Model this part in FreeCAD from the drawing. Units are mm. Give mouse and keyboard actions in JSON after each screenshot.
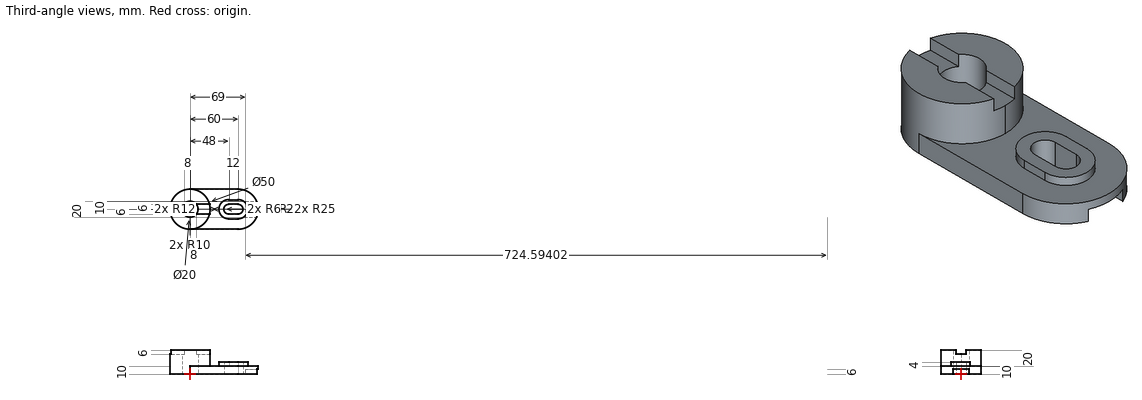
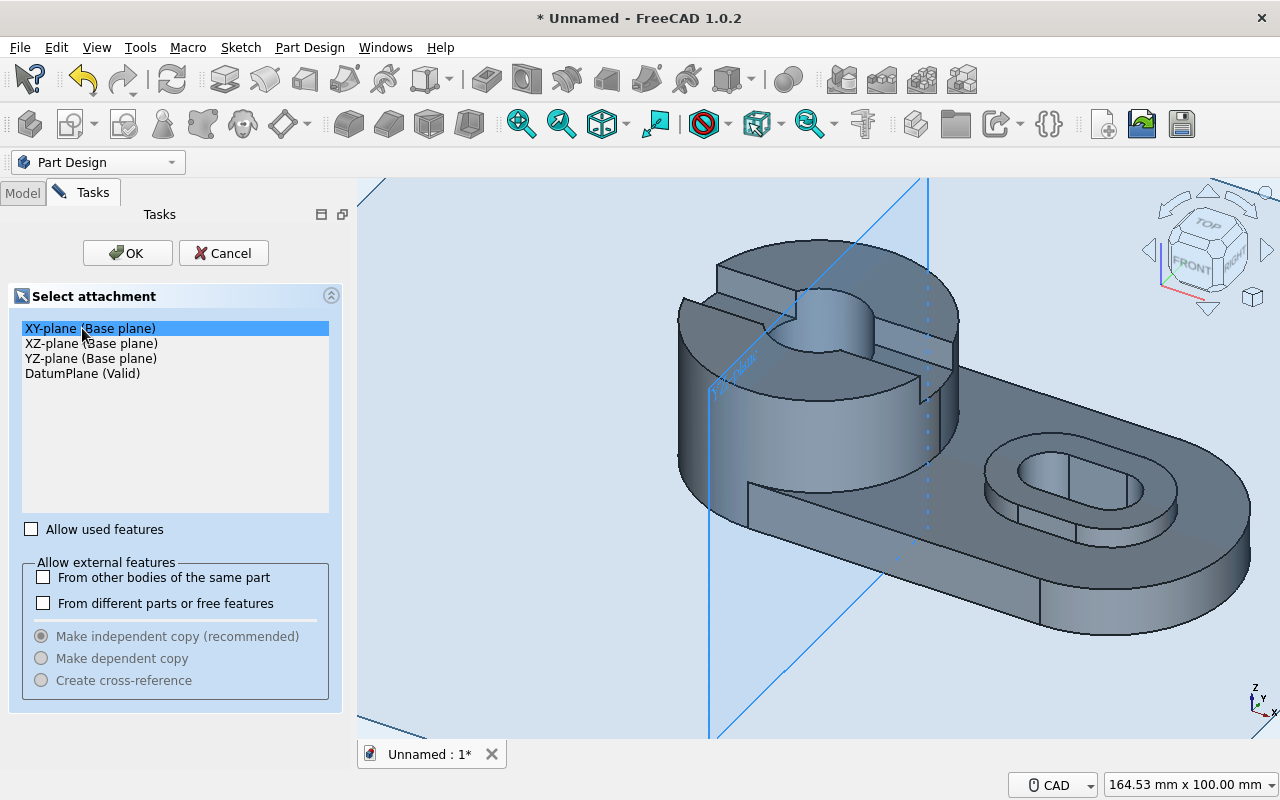
{"action": "left_click", "coordinate": [128, 253]}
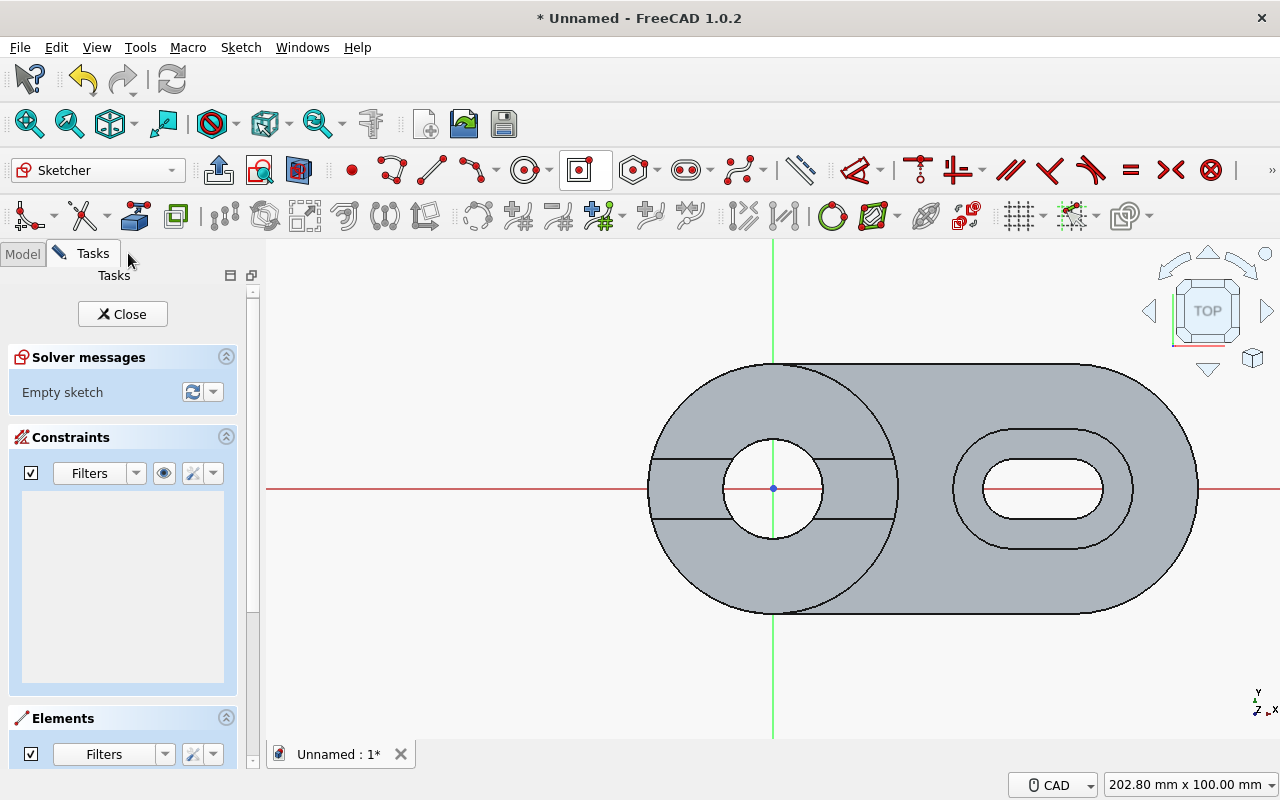
{"action": "left_click", "coordinate": [300, 170]}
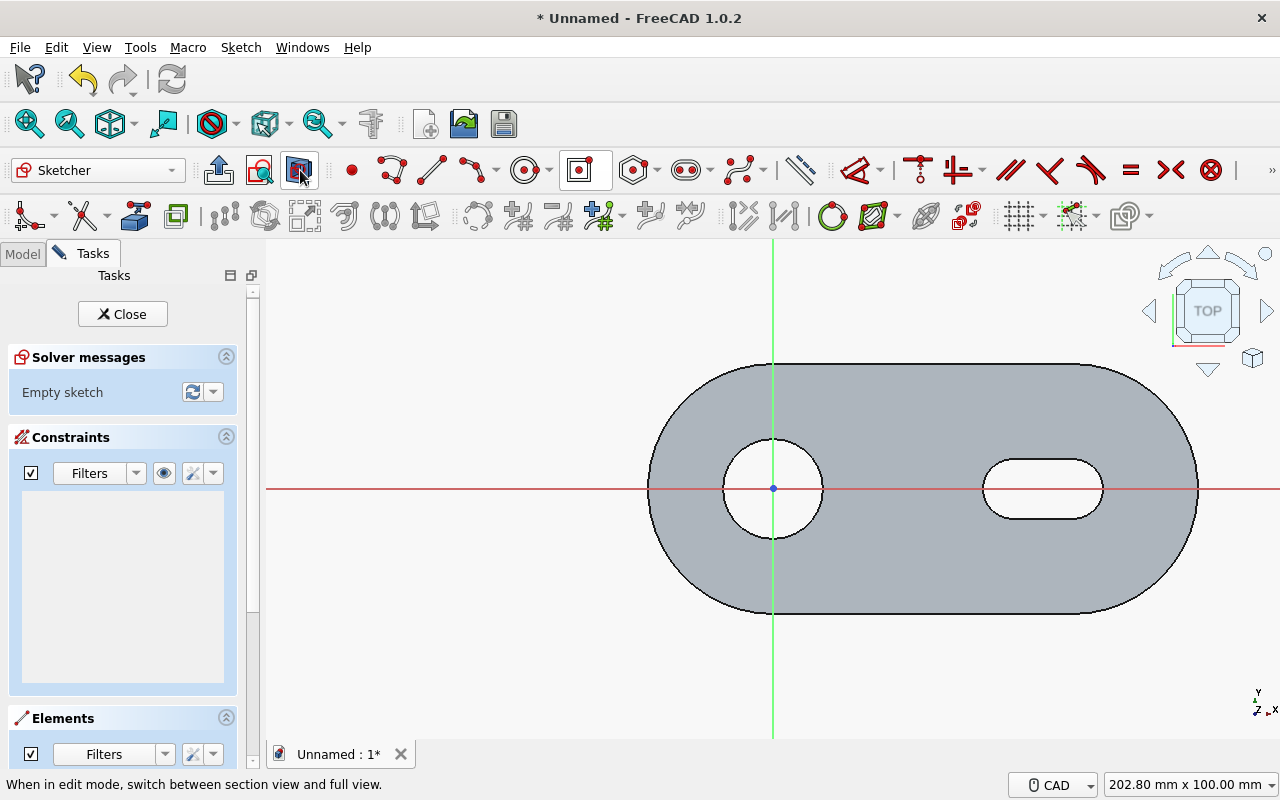
{"action": "scroll", "coordinate": [383, 489], "scroll_direction": "down", "scroll_amount": 10}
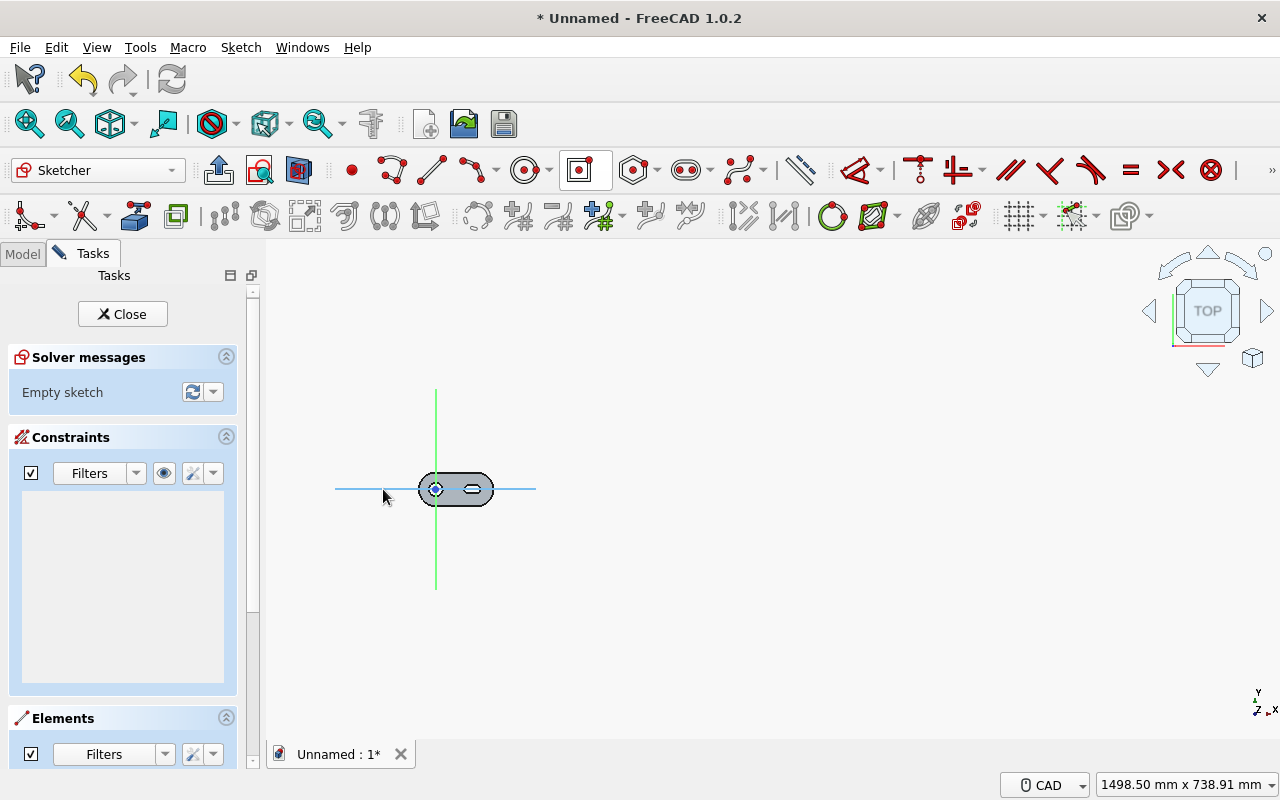
{"action": "key", "text": "g r"}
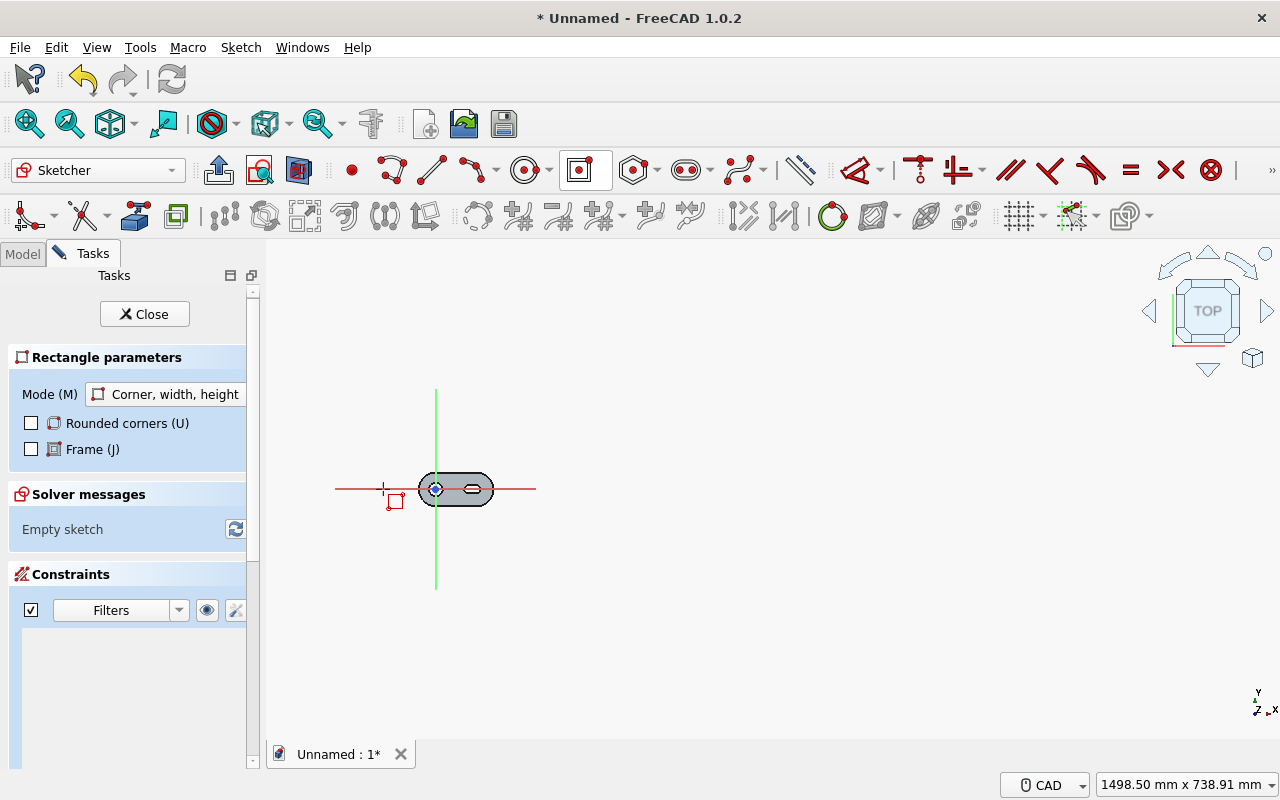
{"action": "scroll", "coordinate": [483, 483], "scroll_direction": "up", "scroll_amount": 5}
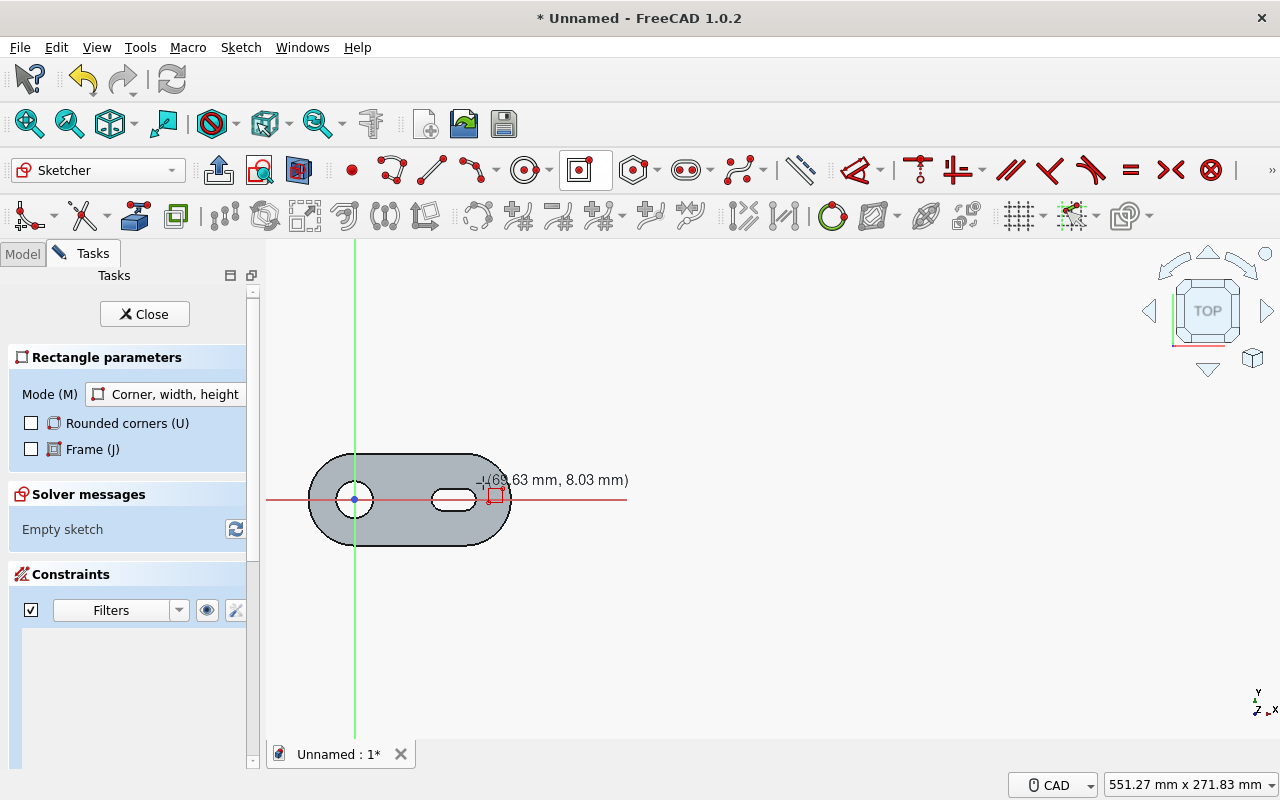
{"action": "left_click", "coordinate": [481, 481]}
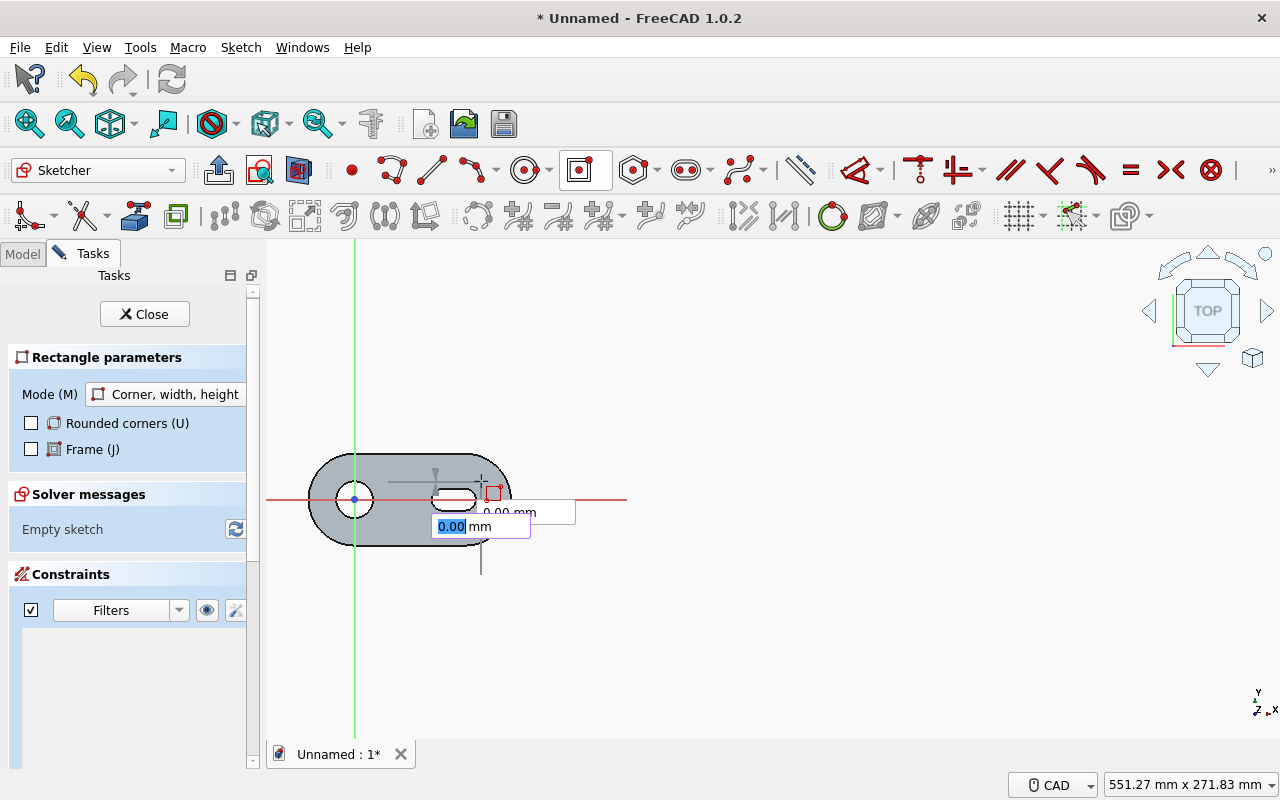
{"action": "scroll", "coordinate": [483, 483], "scroll_direction": "down", "scroll_amount": 5}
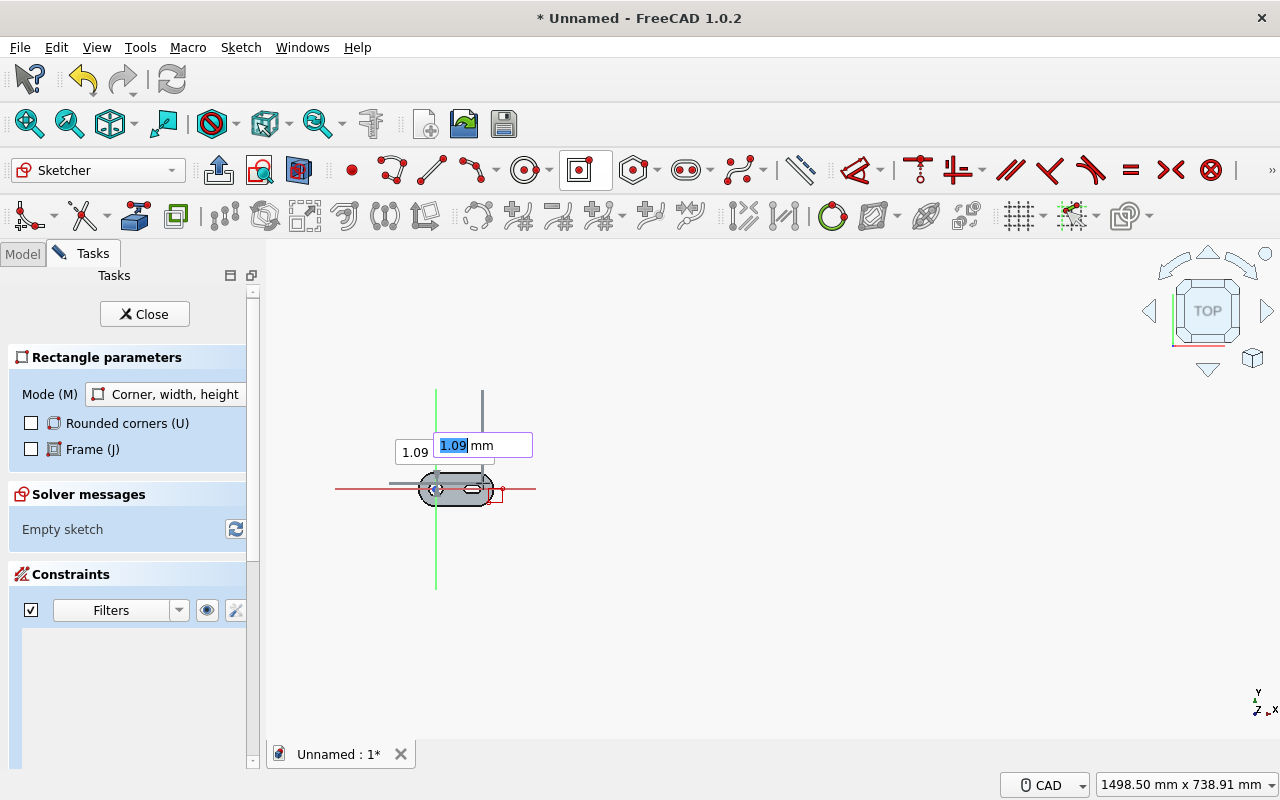
{"action": "scroll", "coordinate": [973, 496], "scroll_direction": "up", "scroll_amount": 5}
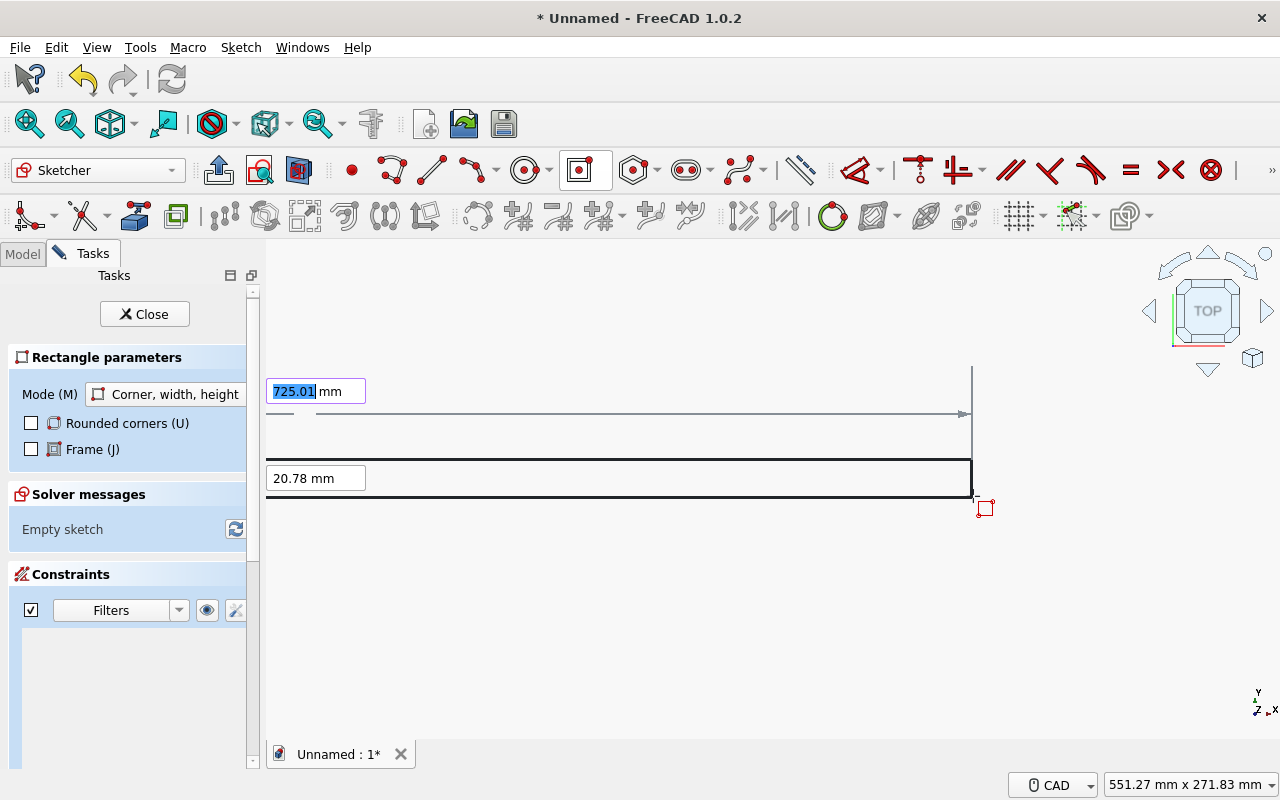
{"action": "left_click", "coordinate": [971, 496]}
{"action": "key", "text": "Escape"}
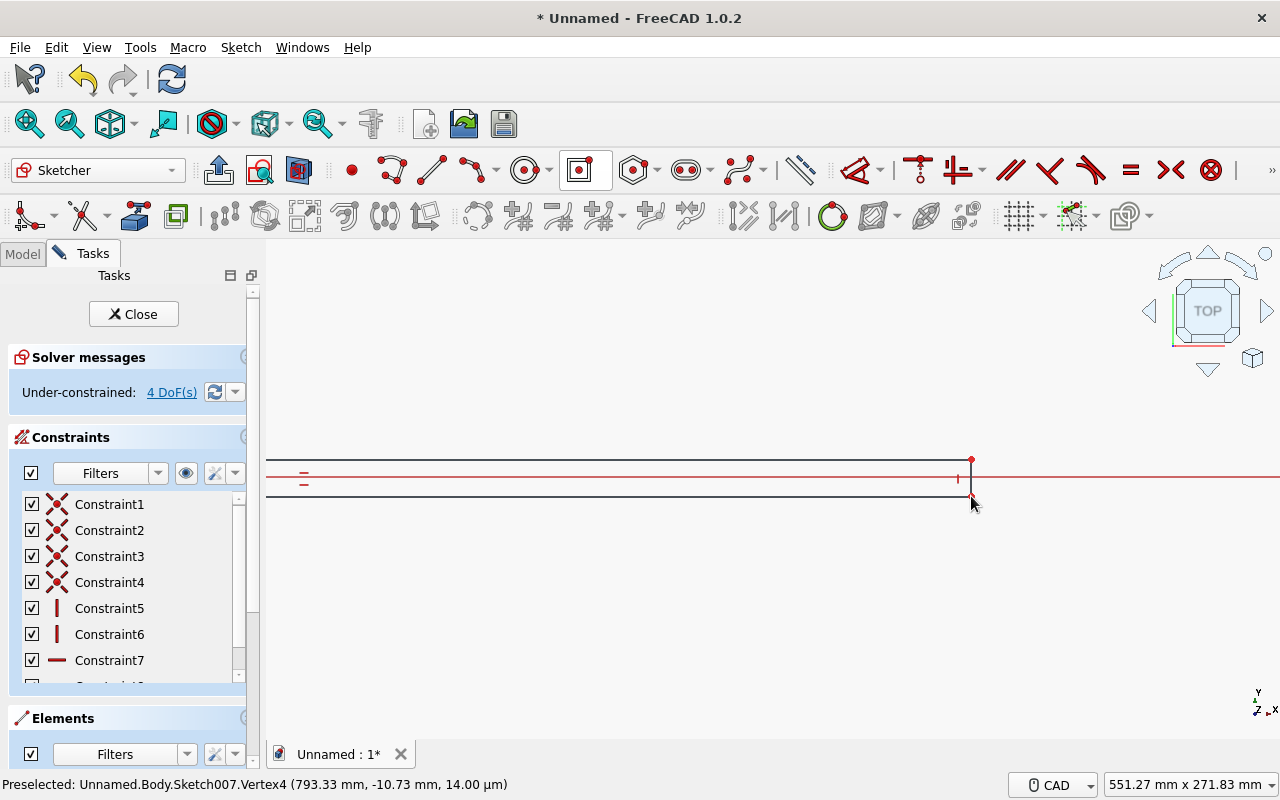
{"action": "left_click", "coordinate": [856, 170]}